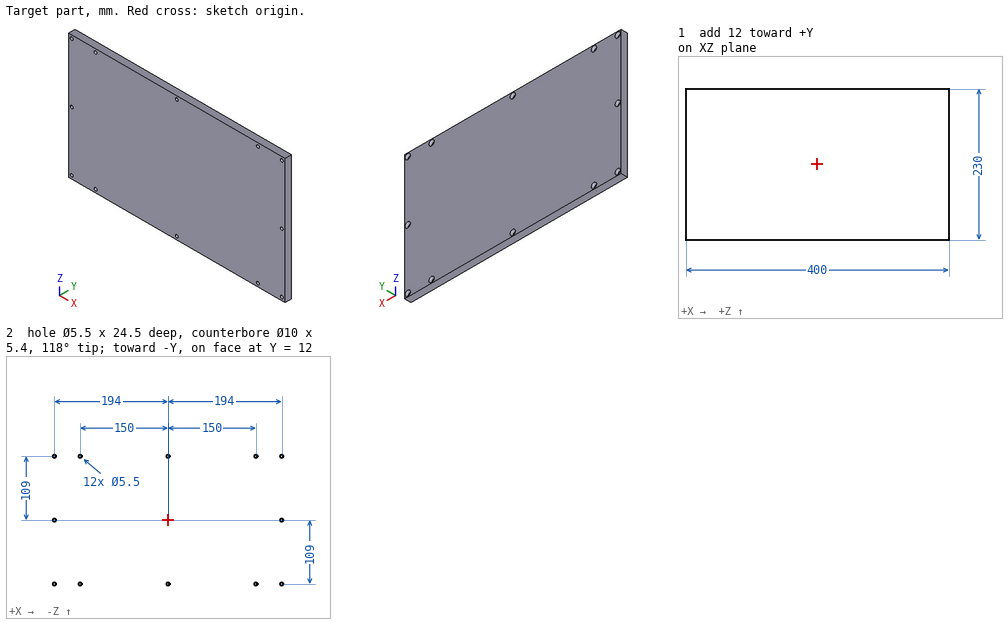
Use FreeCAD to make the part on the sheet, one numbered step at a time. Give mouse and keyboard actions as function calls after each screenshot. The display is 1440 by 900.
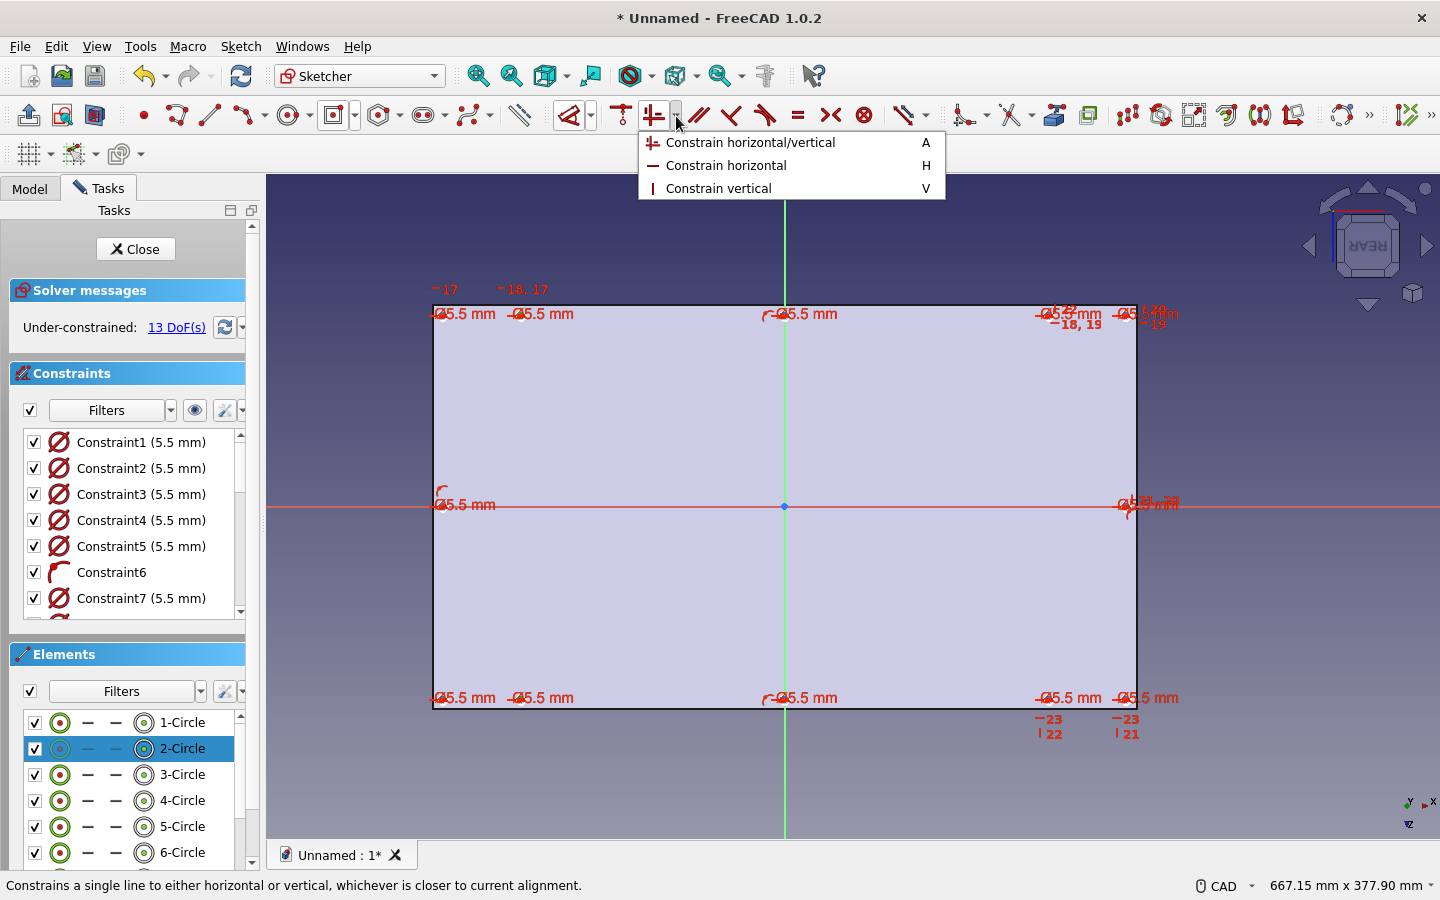
click(792, 188)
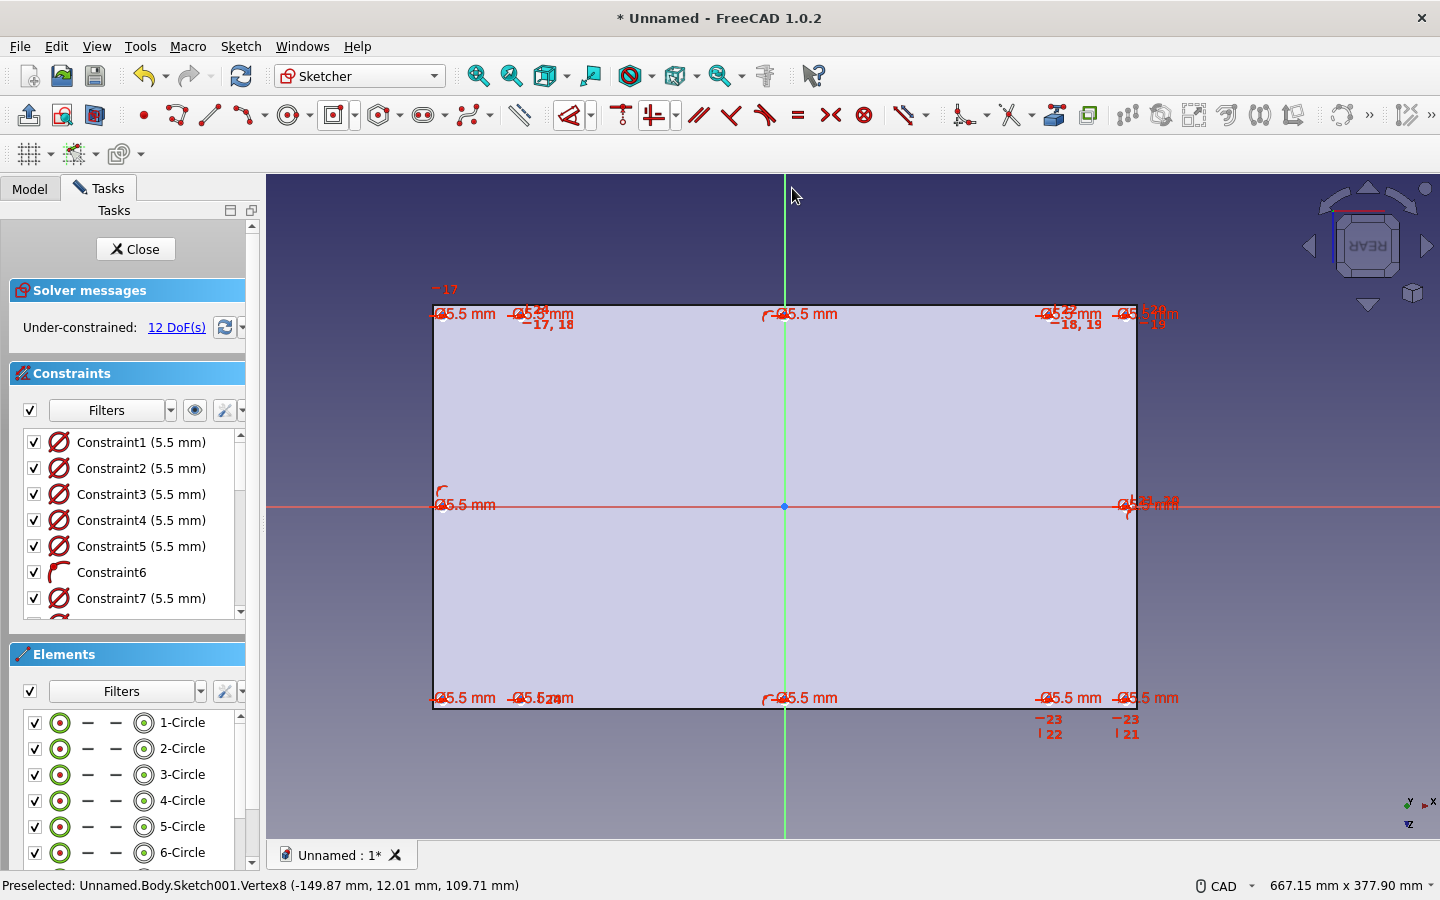
click(1049, 700)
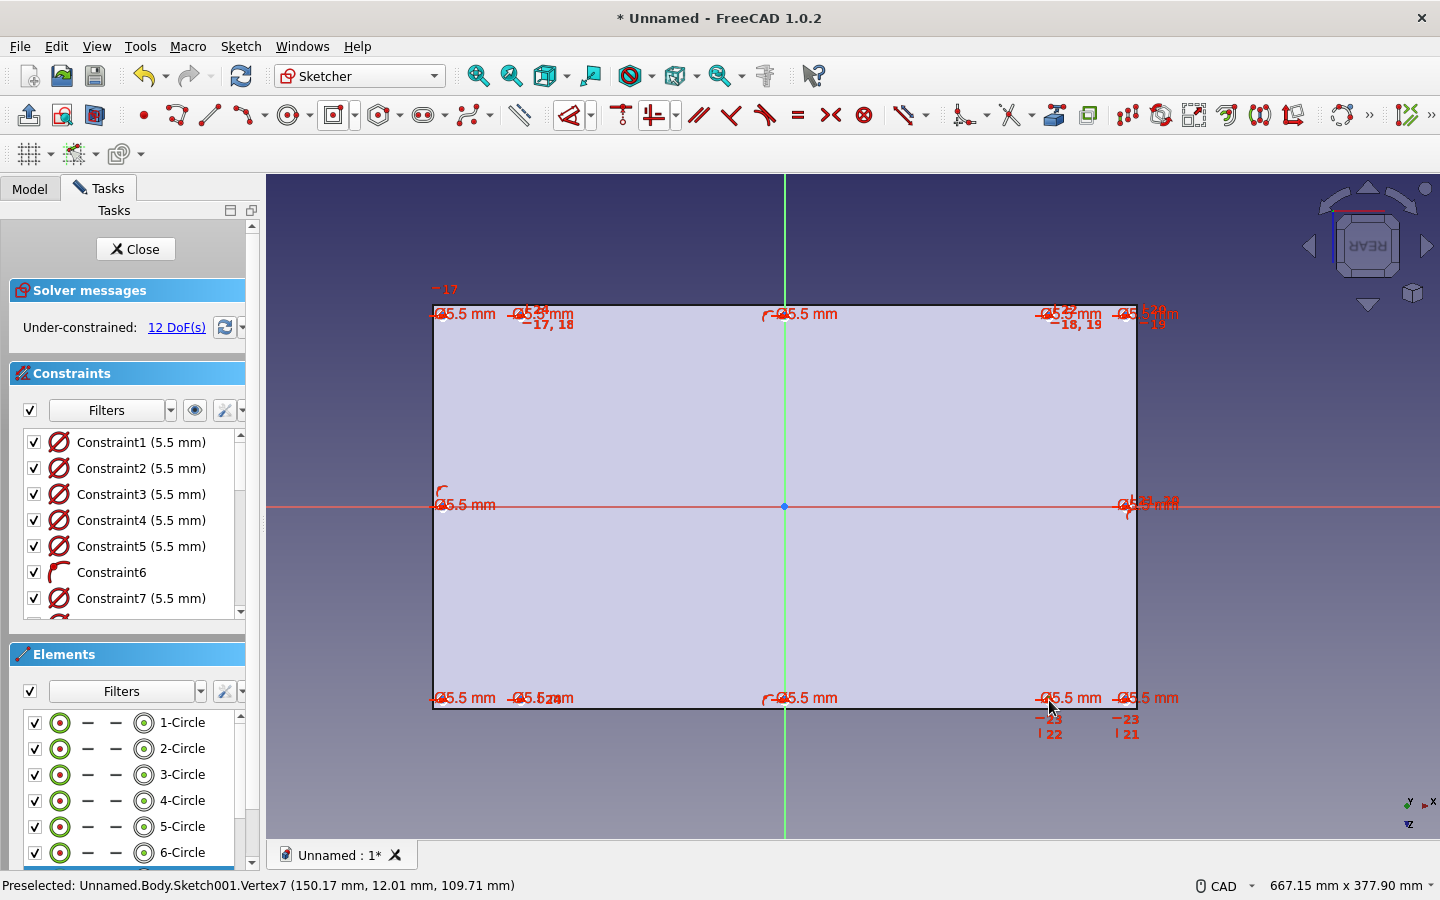
click(521, 700)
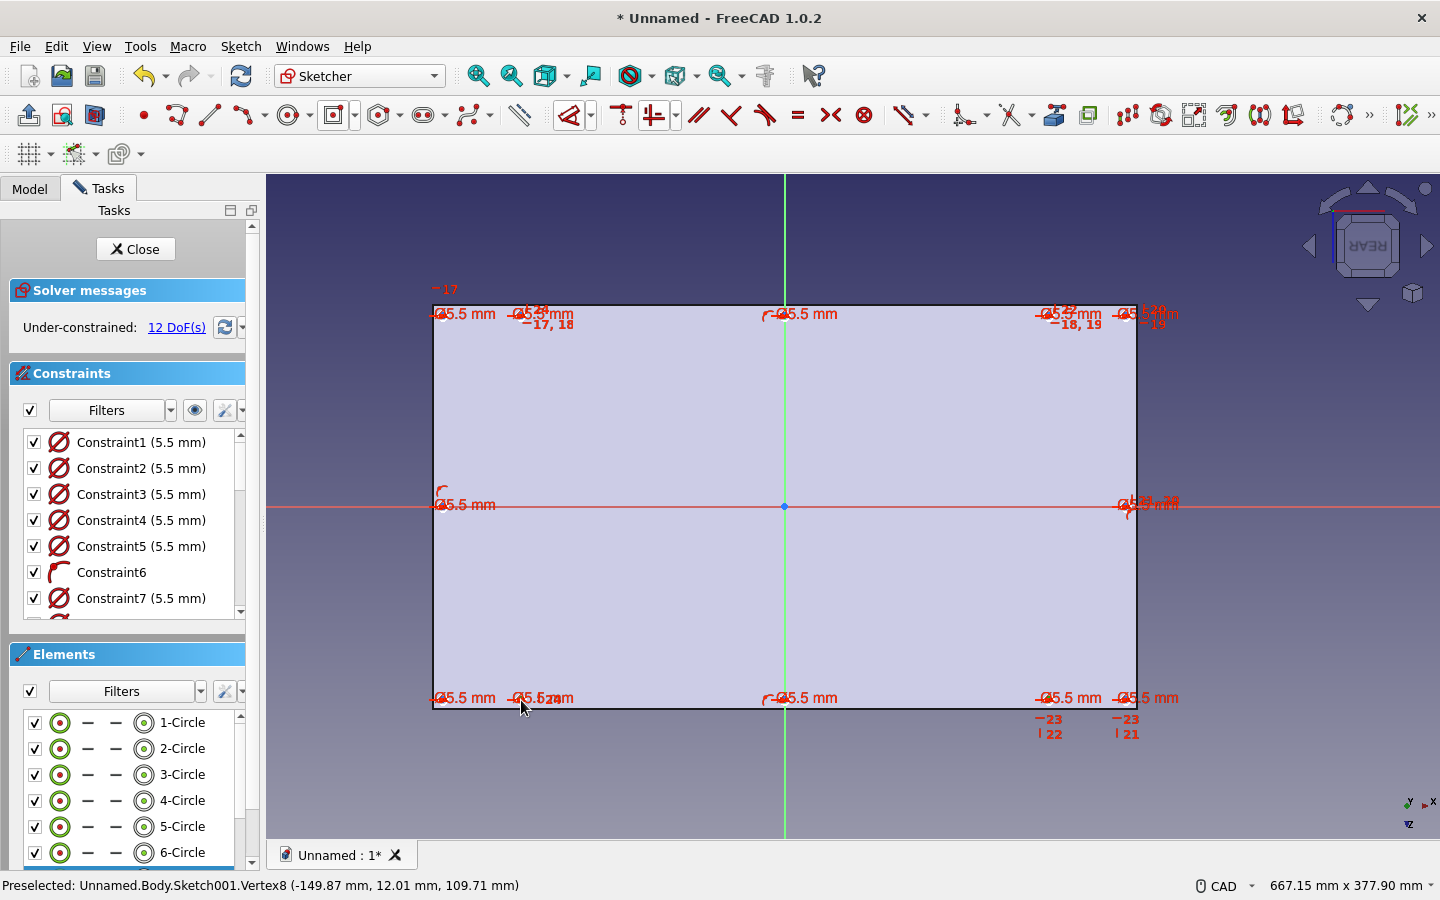
key(h)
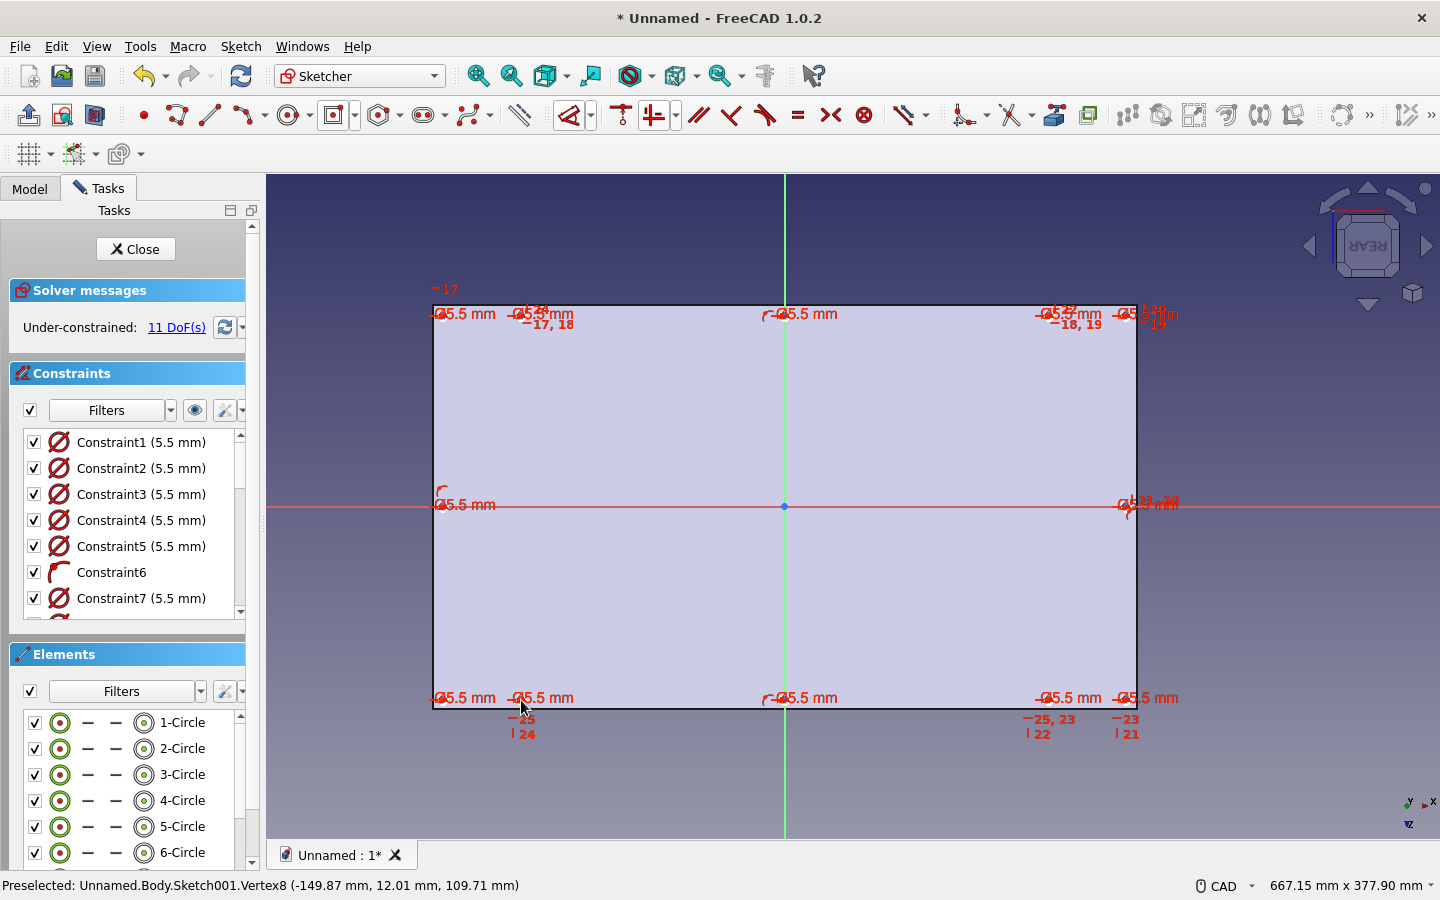
click(443, 316)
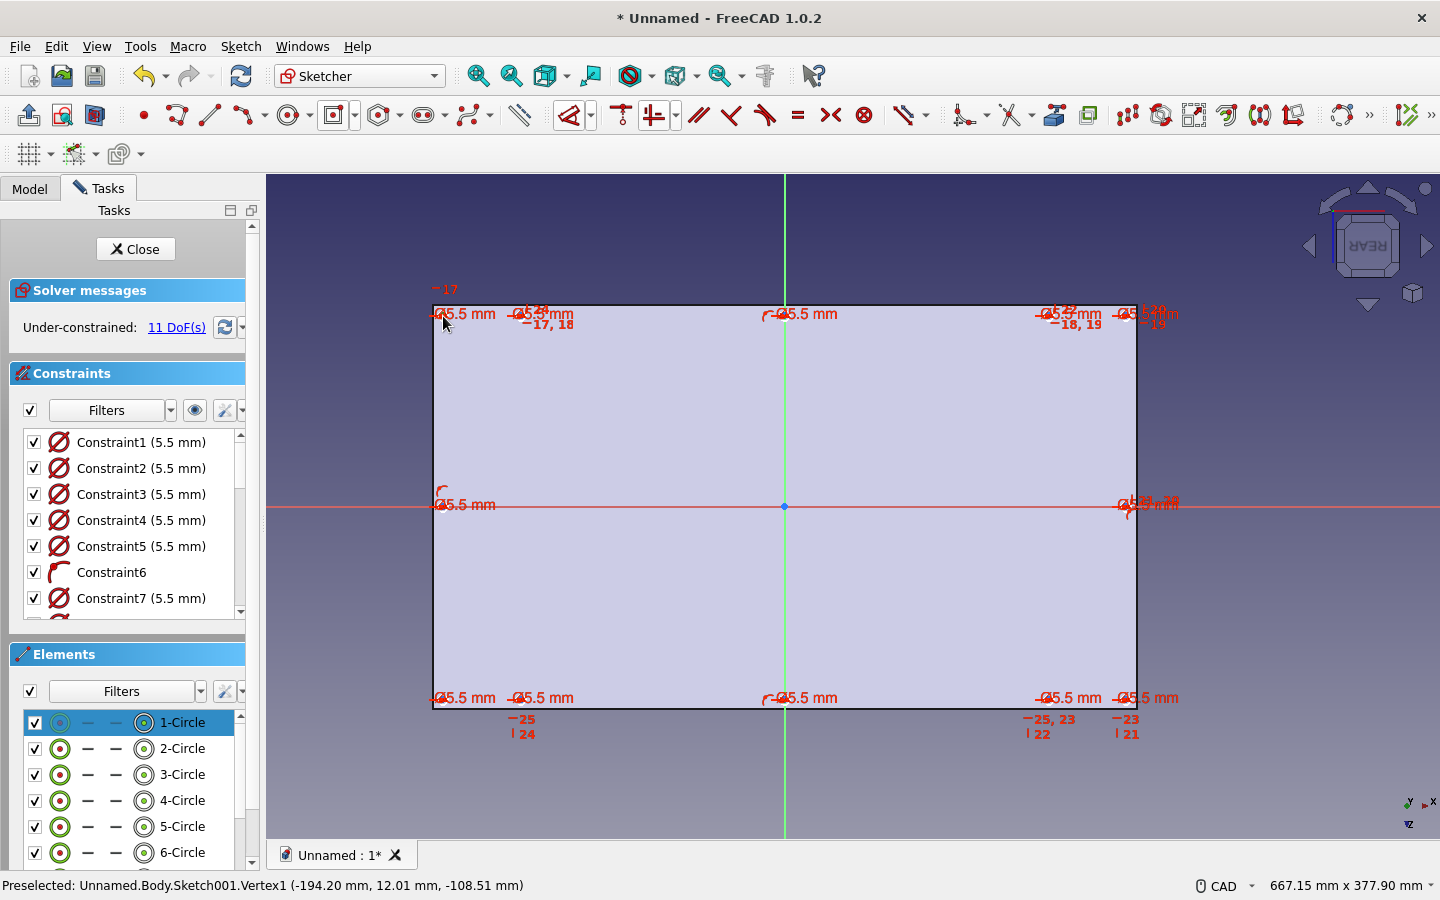
click(443, 700)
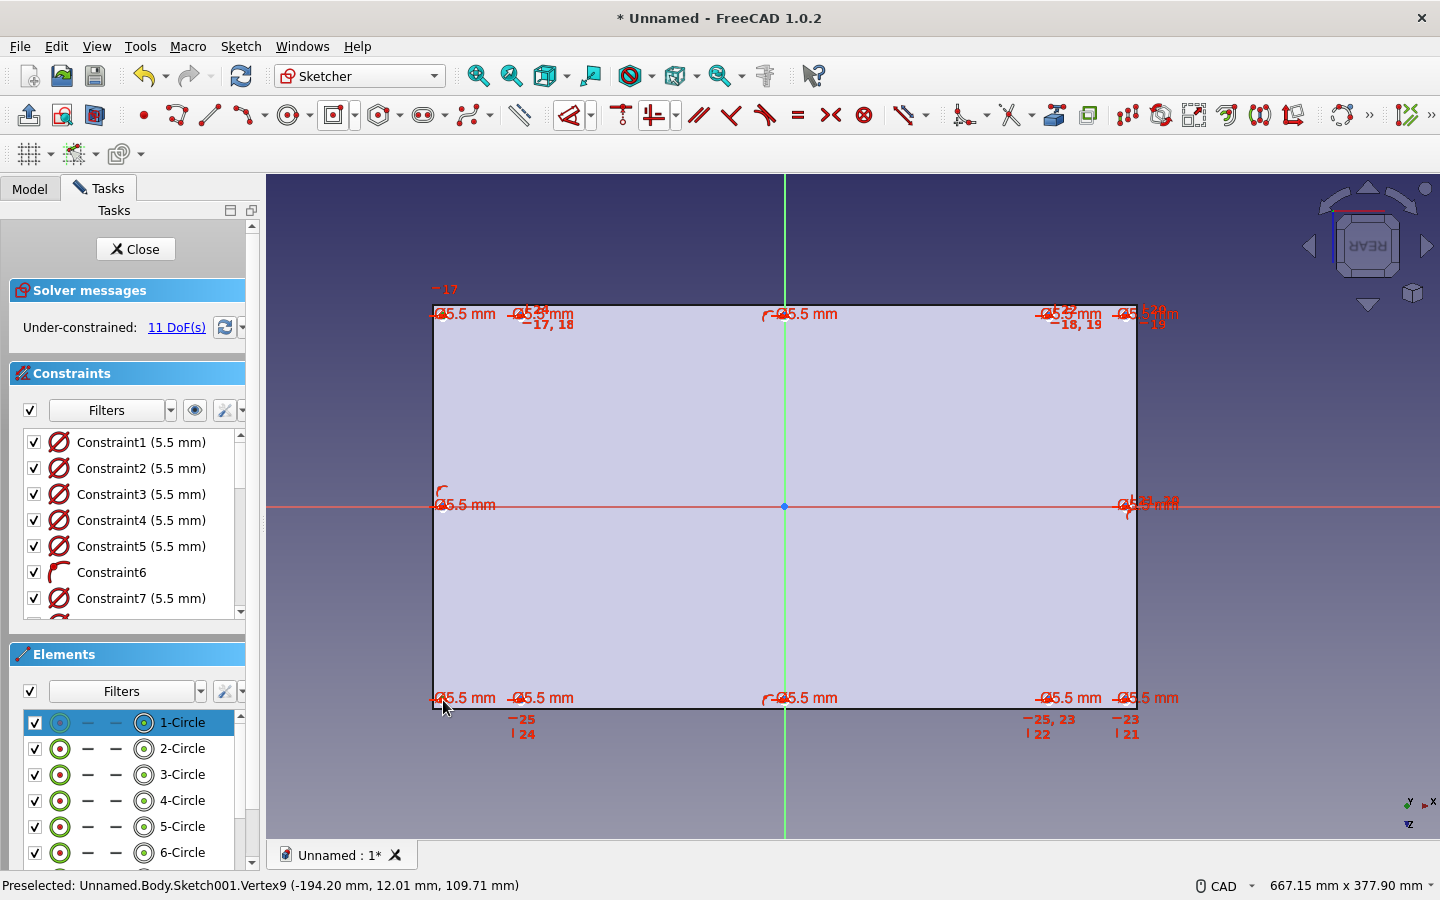
key(v)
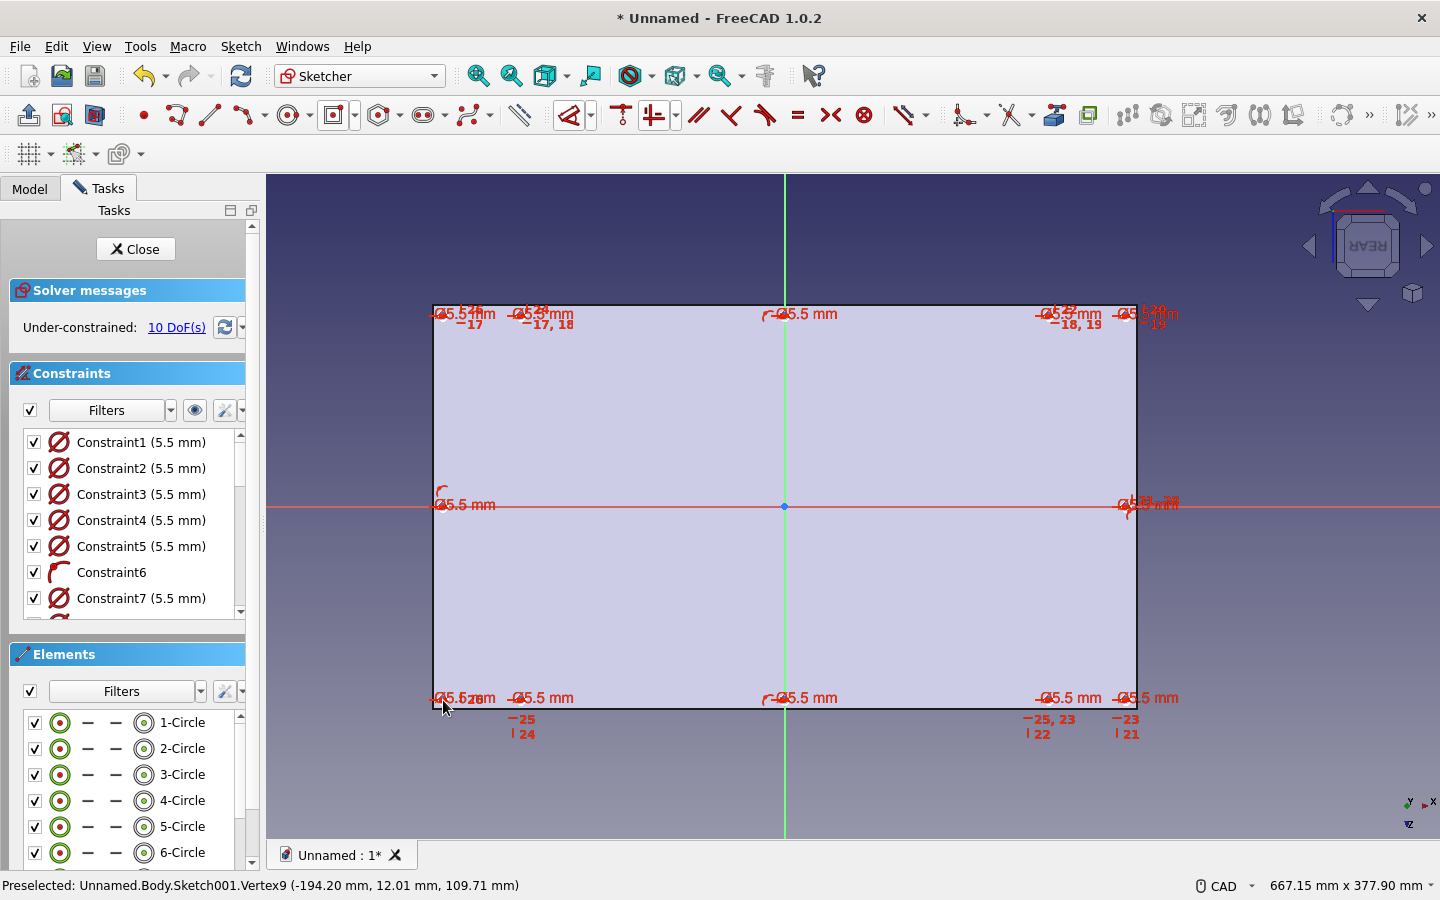
click(521, 700)